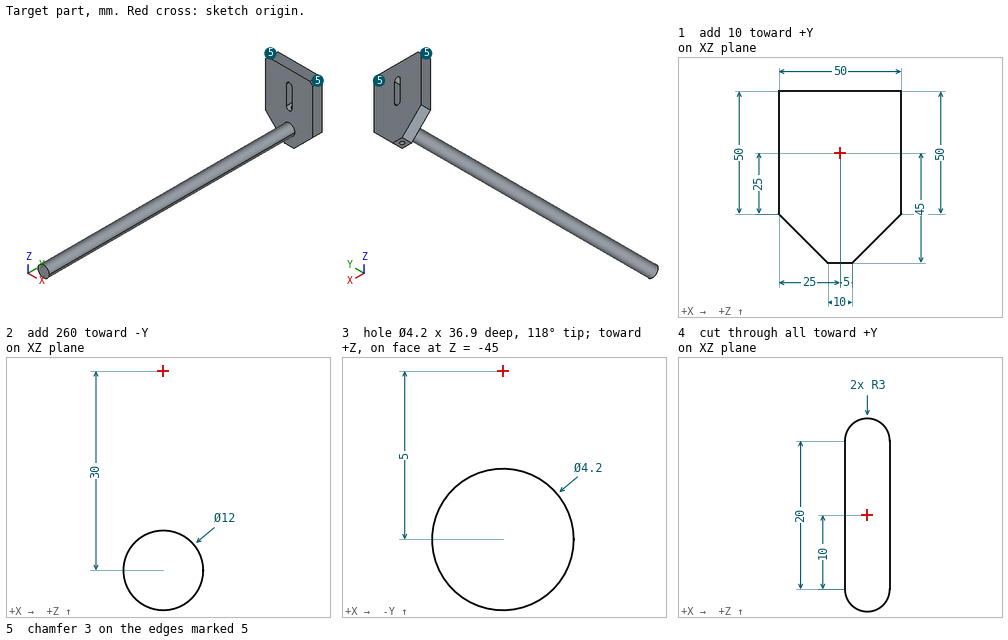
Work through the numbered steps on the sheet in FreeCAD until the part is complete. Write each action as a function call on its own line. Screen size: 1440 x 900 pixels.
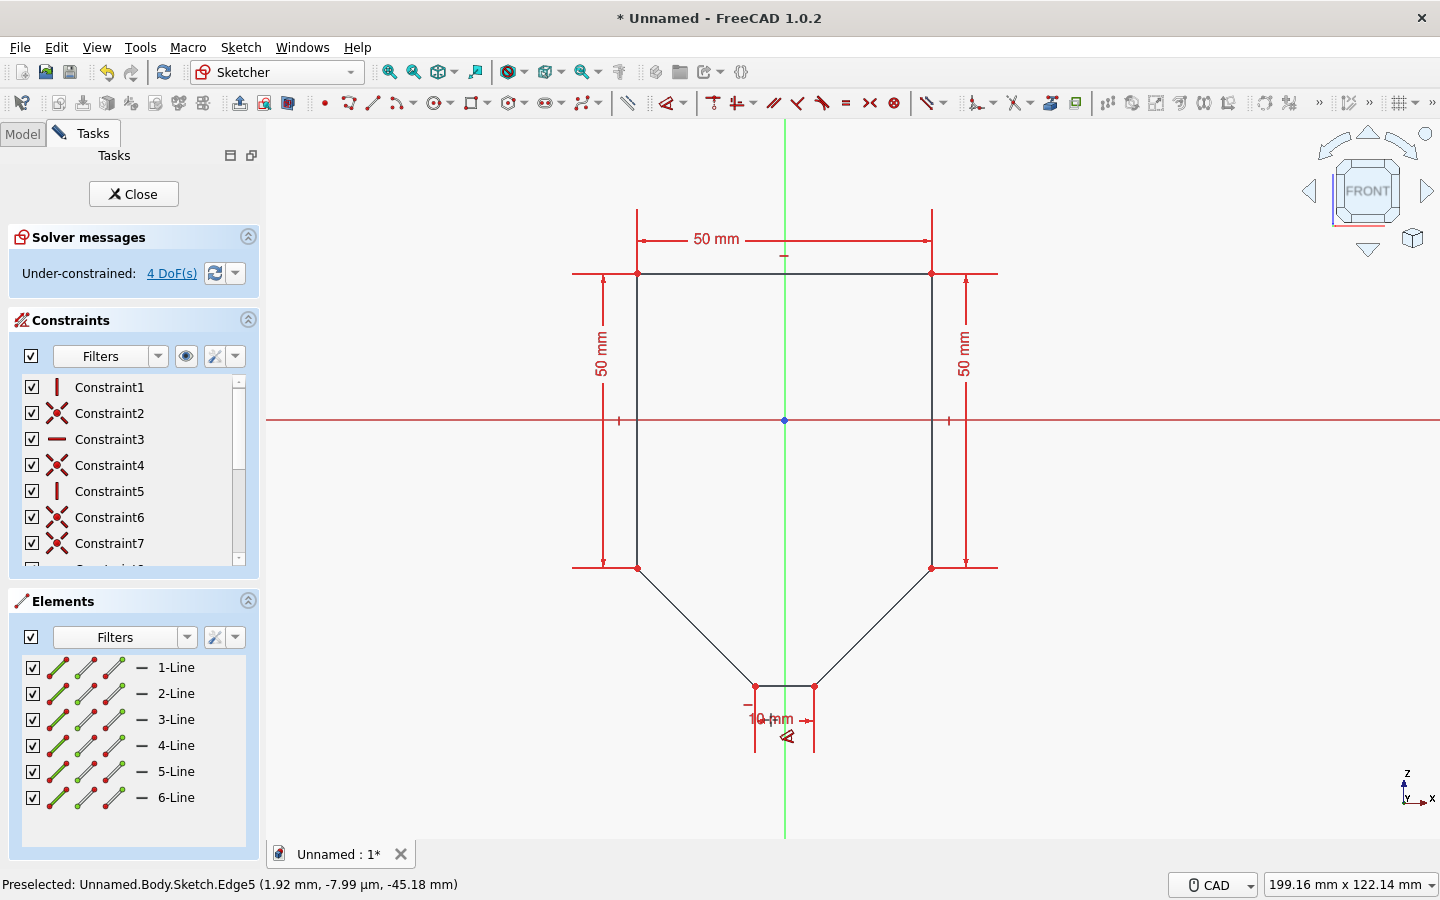
scroll(814, 686, up, 2)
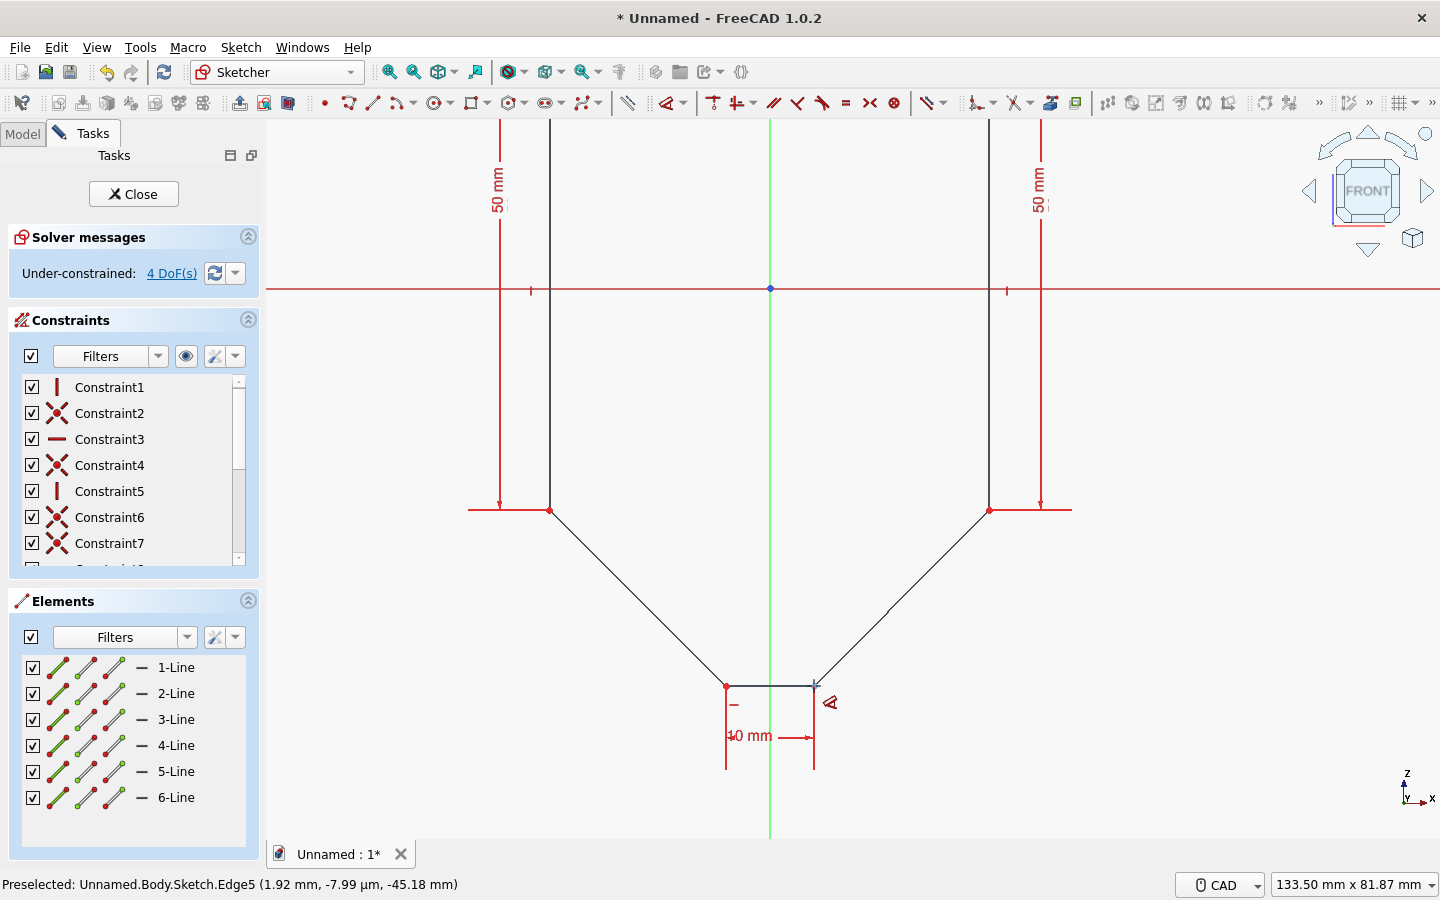
click(814, 686)
click(792, 255)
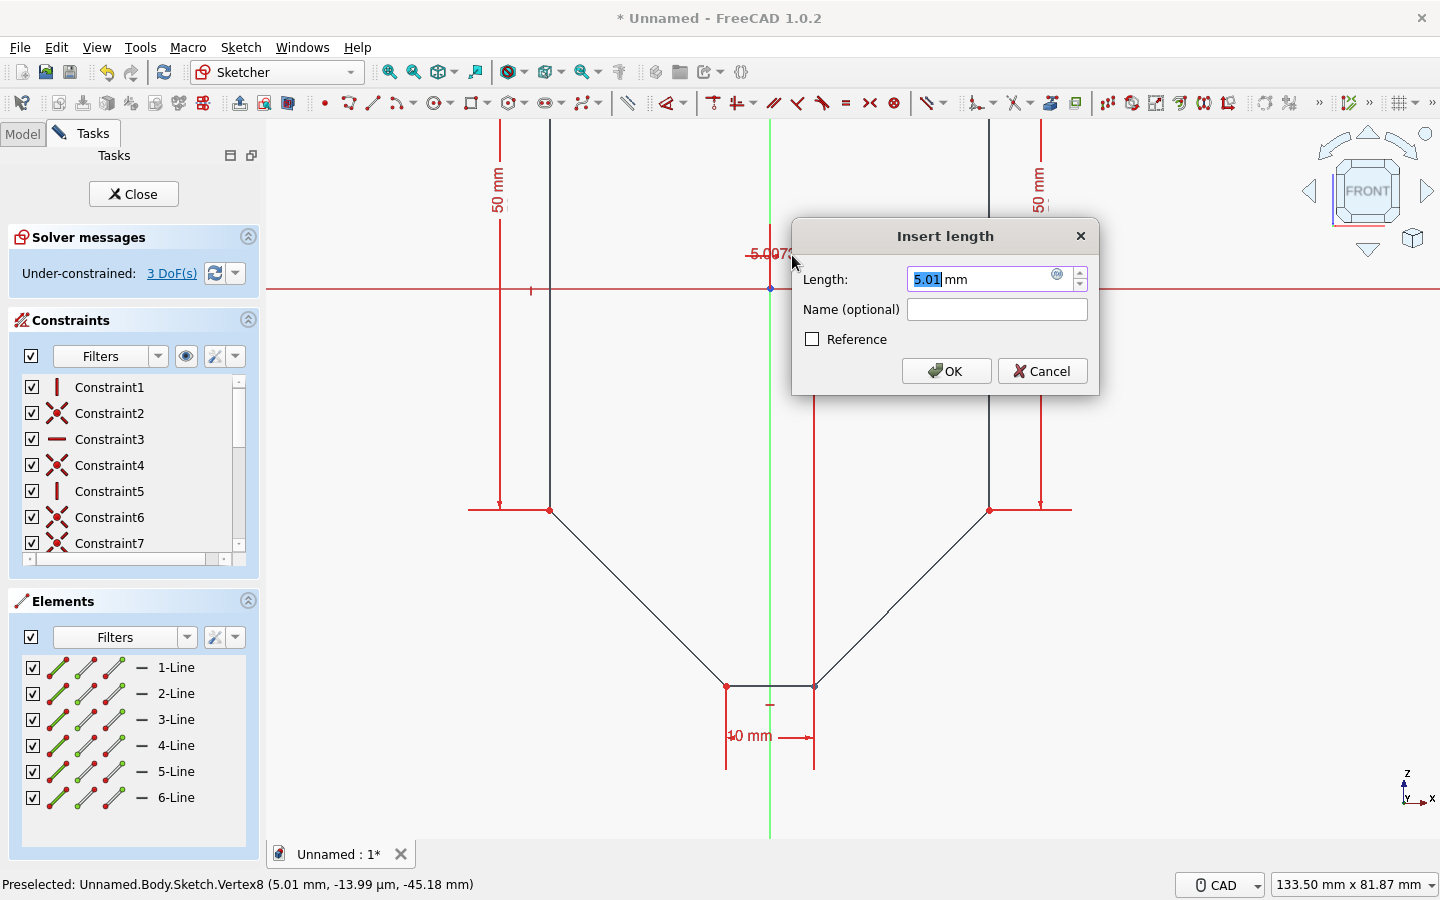
text(5)
key(Return)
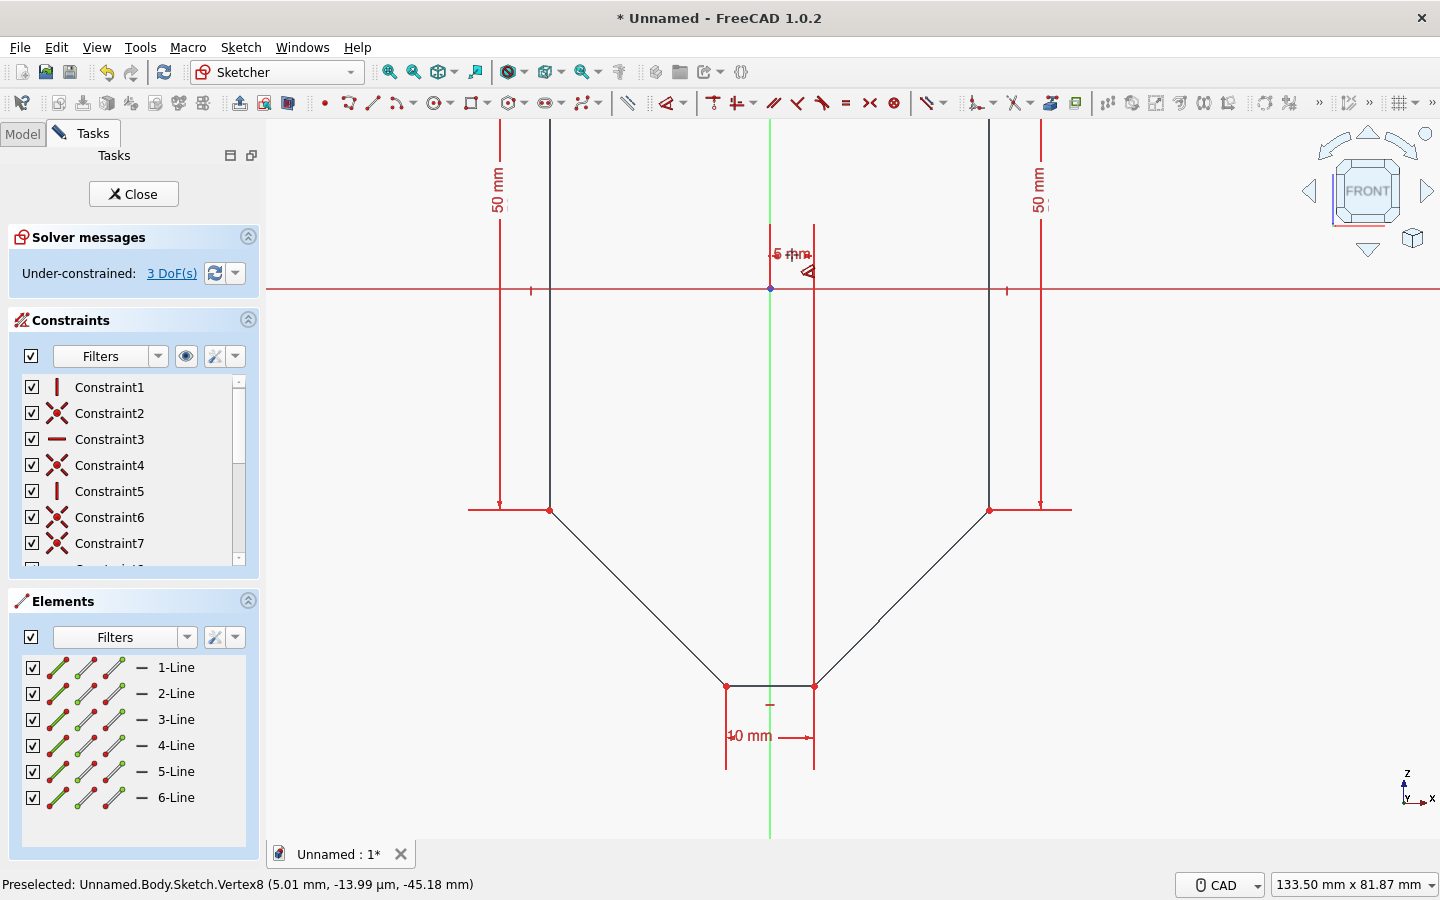
click(550, 510)
click(660, 544)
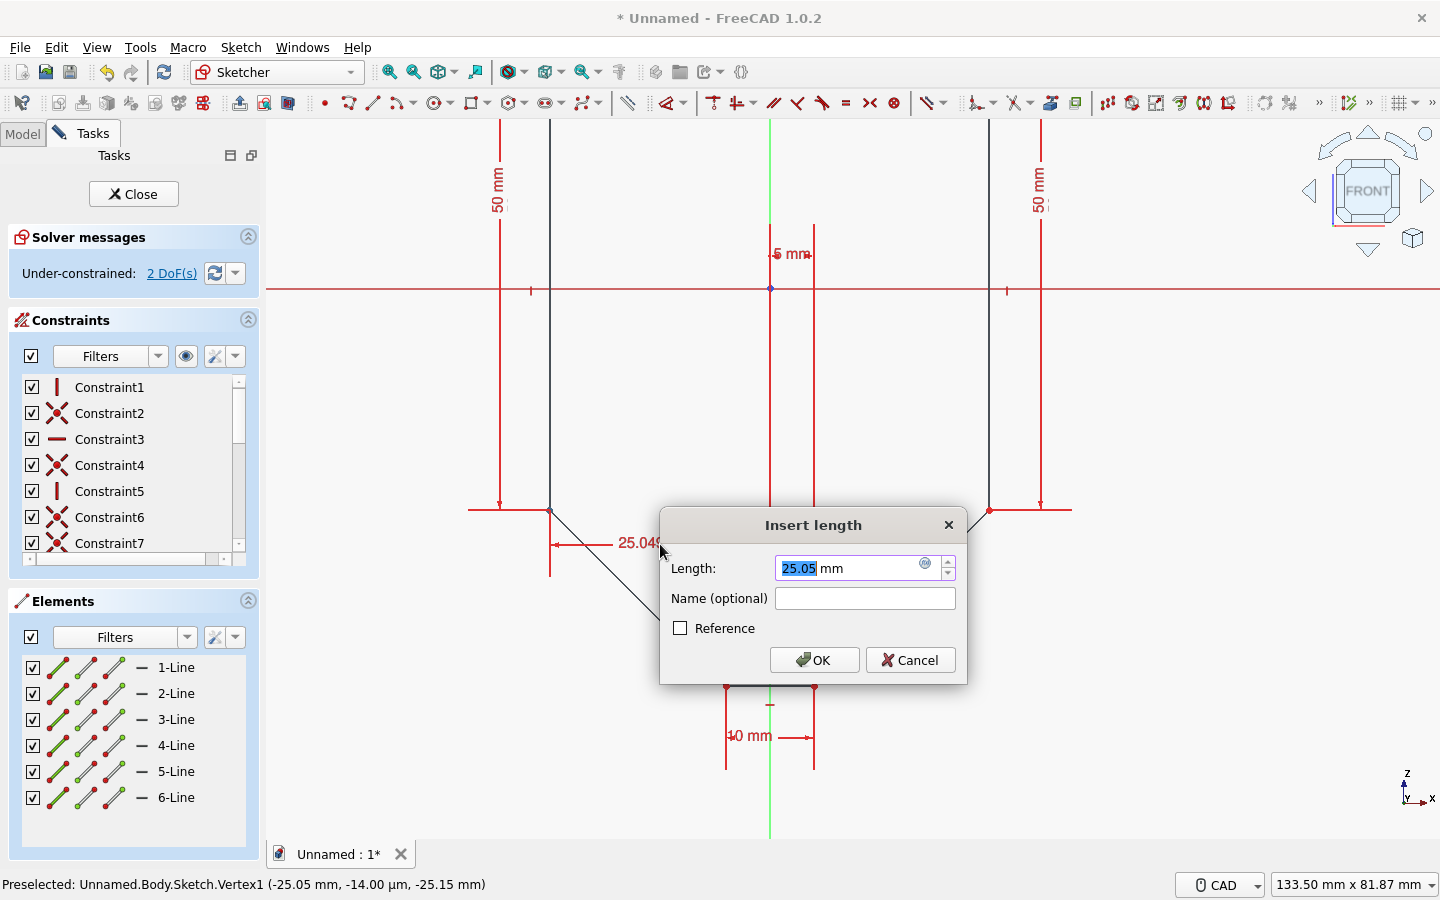
text(25)
key(Return)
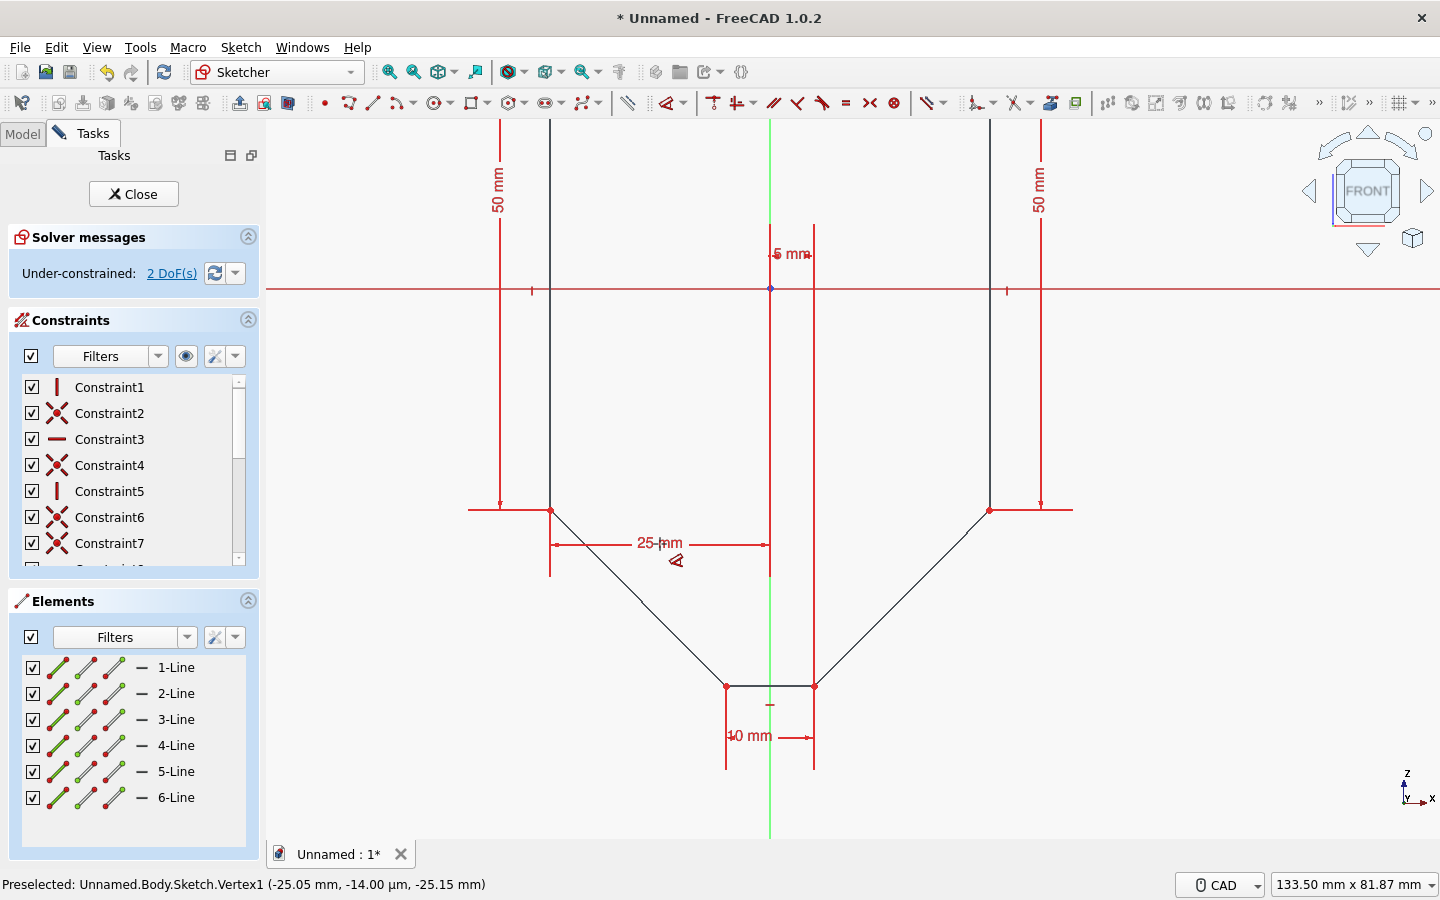
click(550, 510)
click(516, 399)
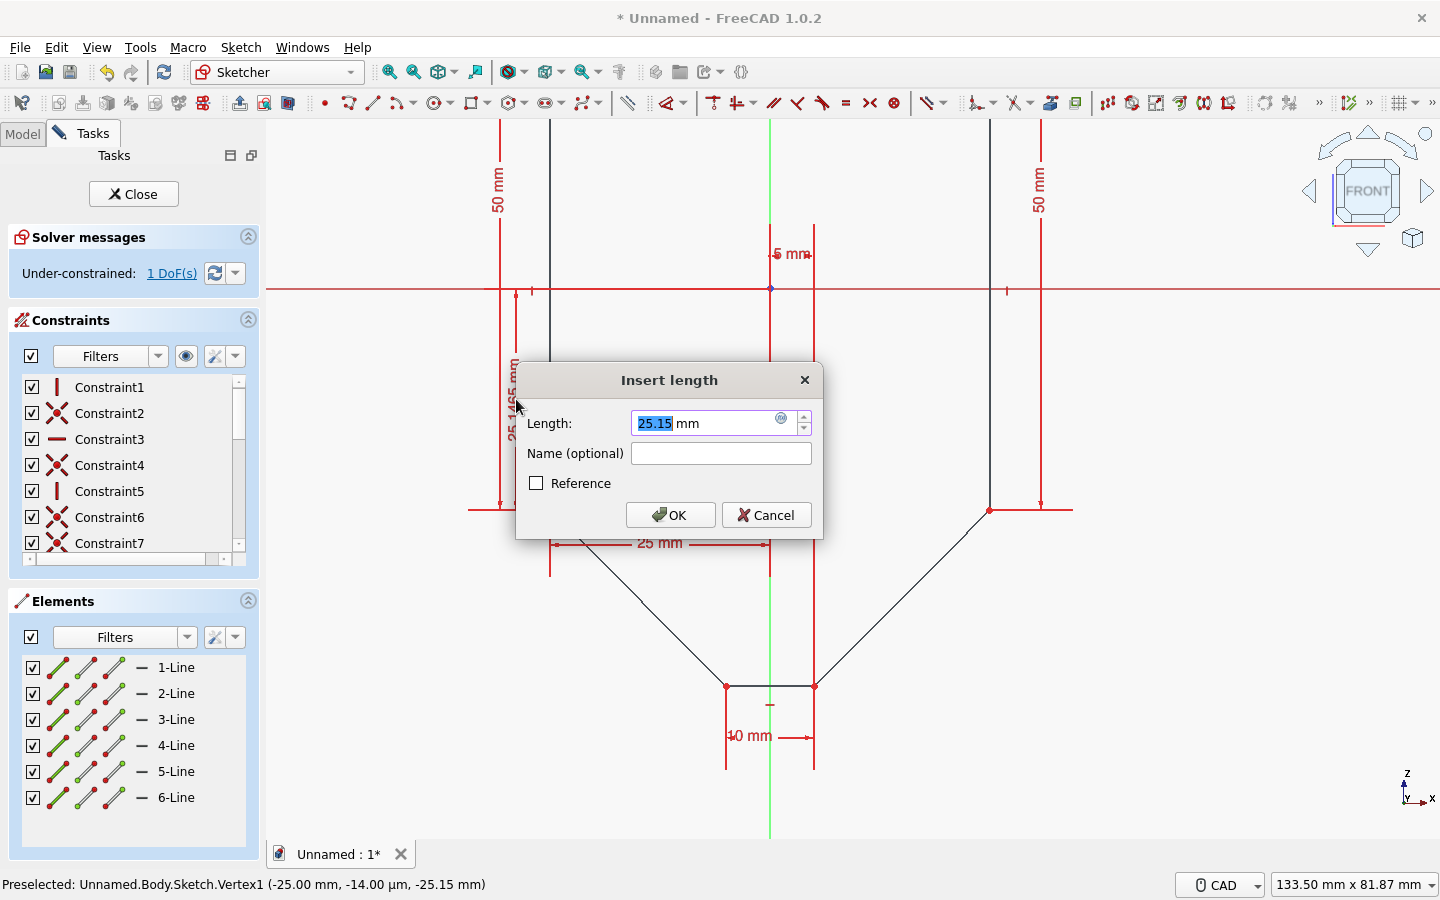
text(25)
key(Return)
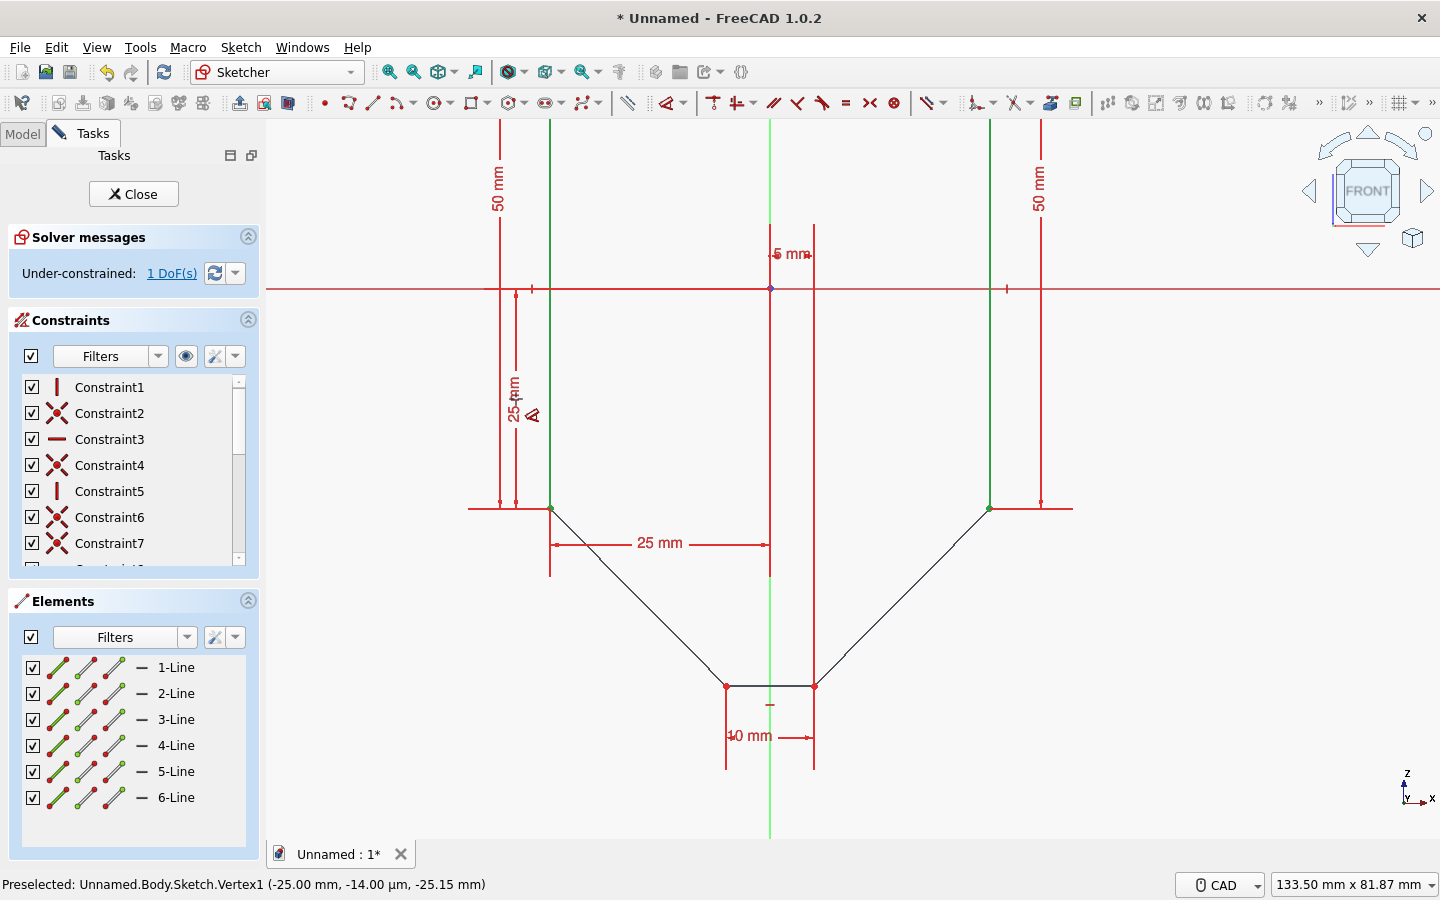
click(814, 686)
click(848, 488)